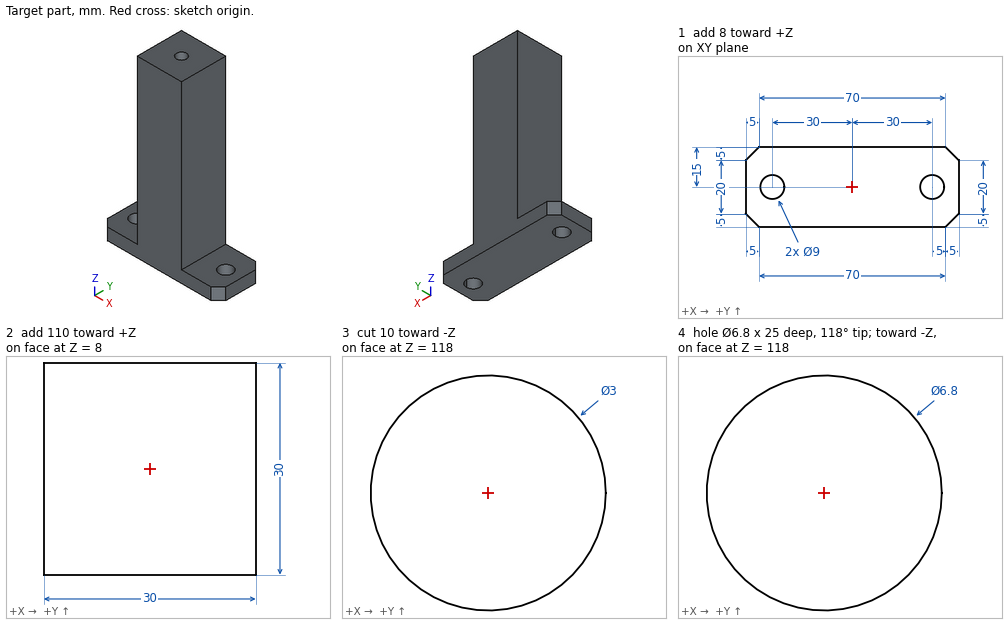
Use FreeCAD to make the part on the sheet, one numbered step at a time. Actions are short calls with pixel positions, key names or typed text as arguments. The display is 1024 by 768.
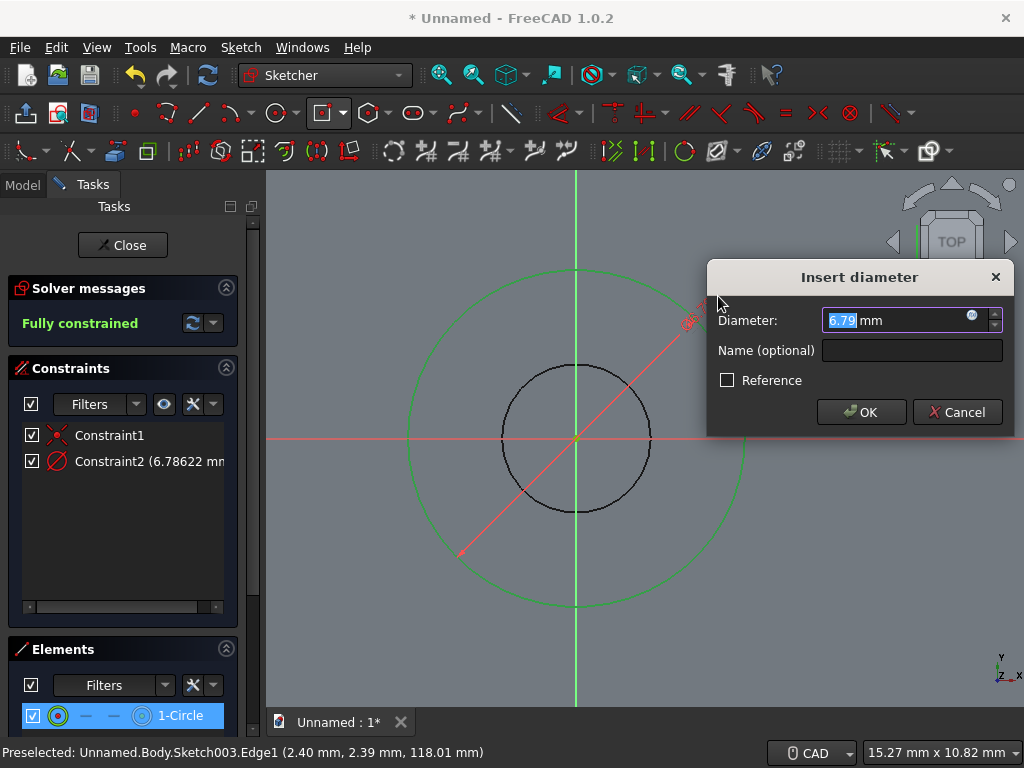
text(6.8)
key(Return)
key(Escape)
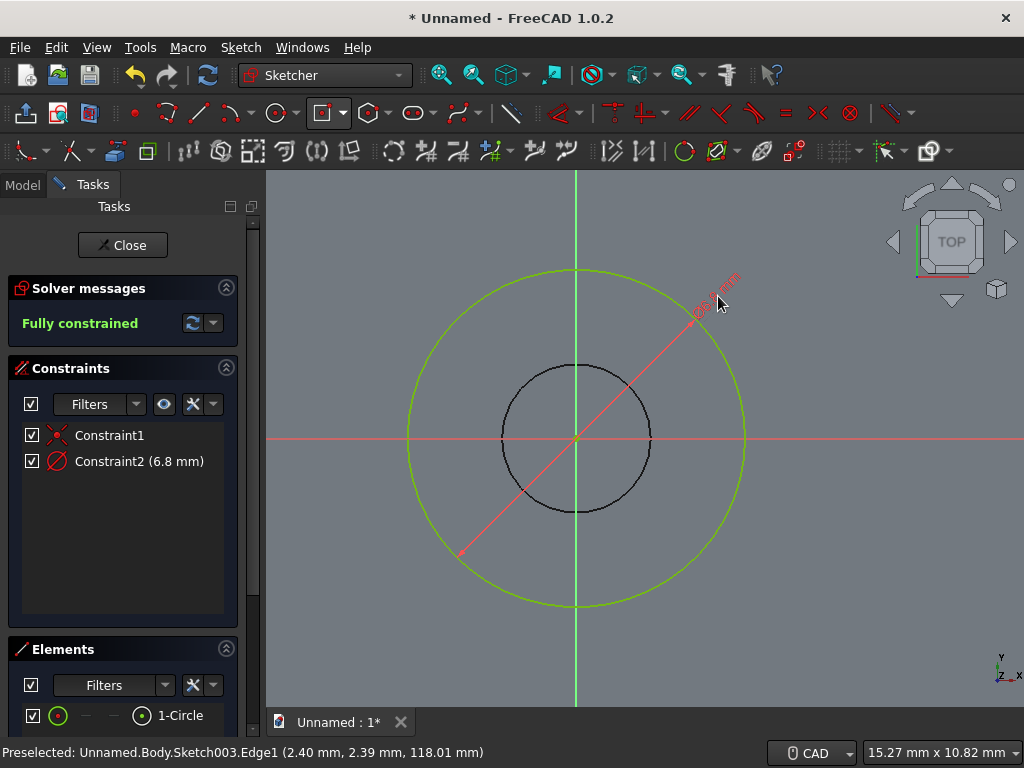
click(123, 245)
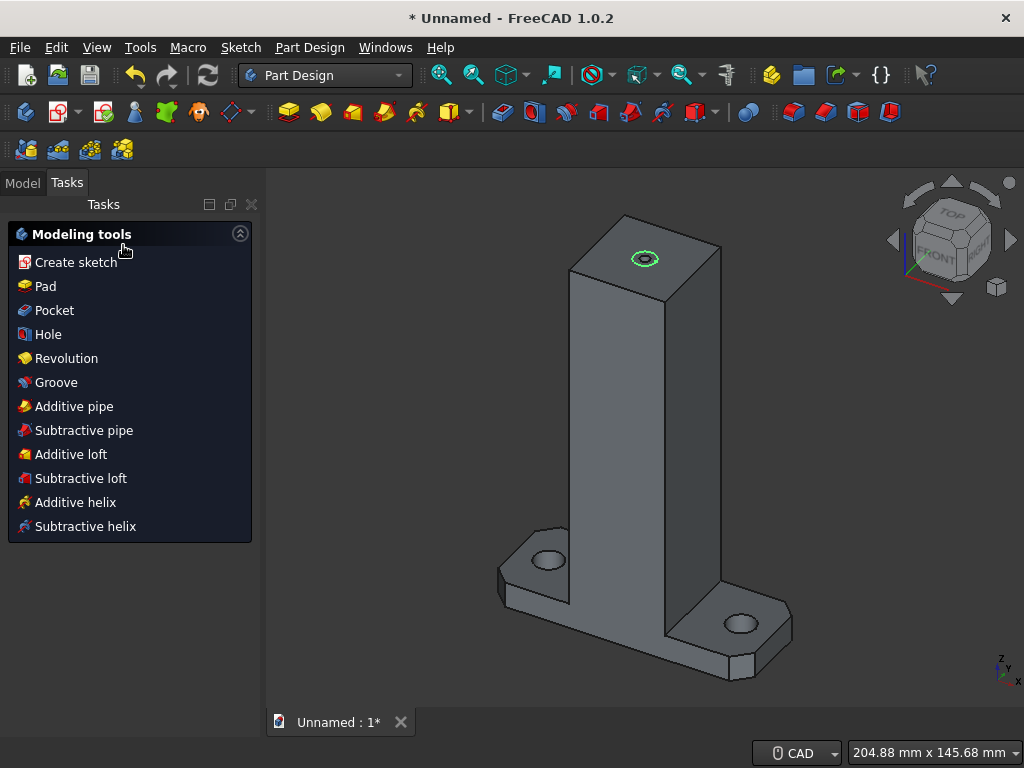
click(536, 112)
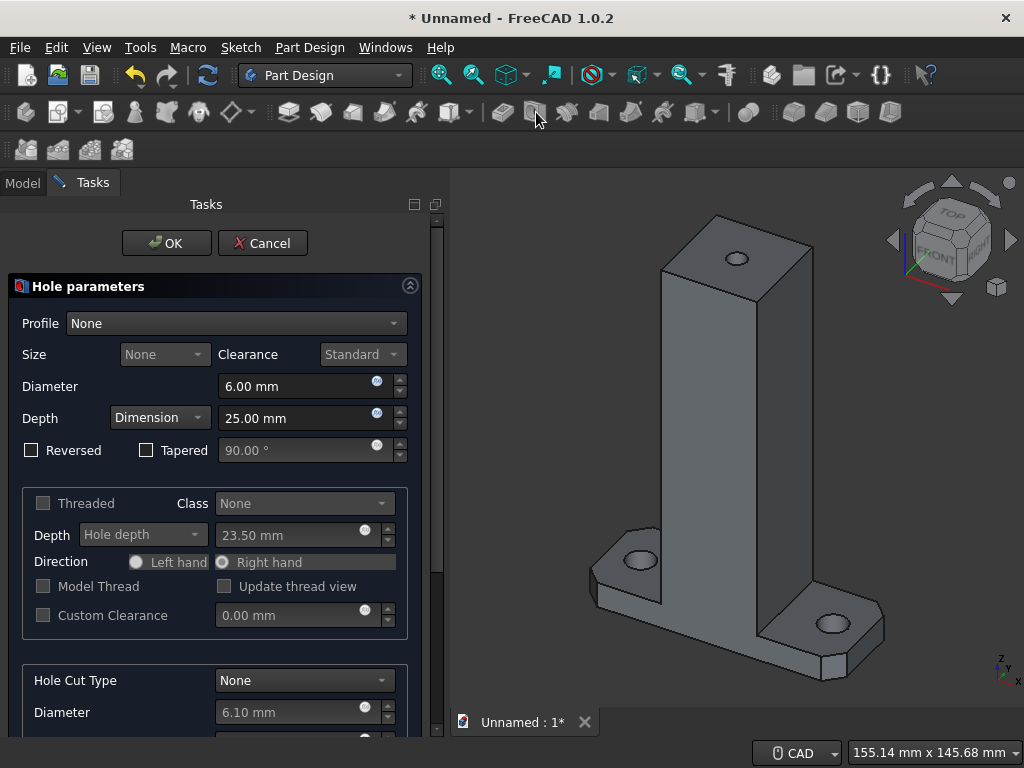
triple_click(305, 386)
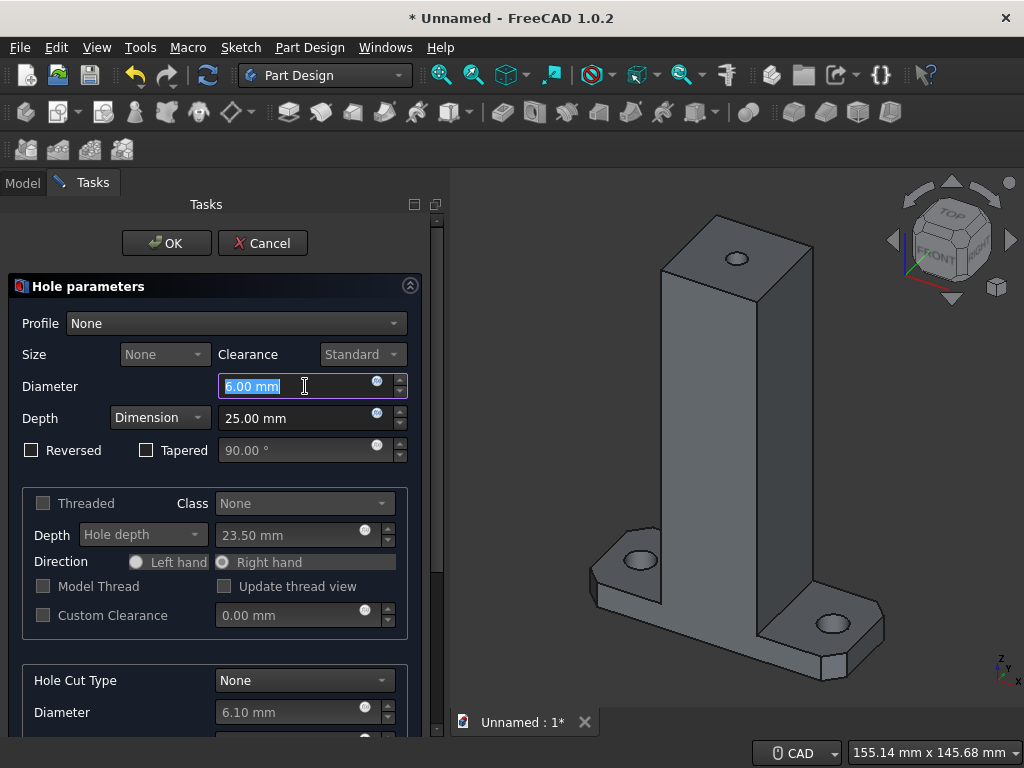
text(6.8)
key(Tab)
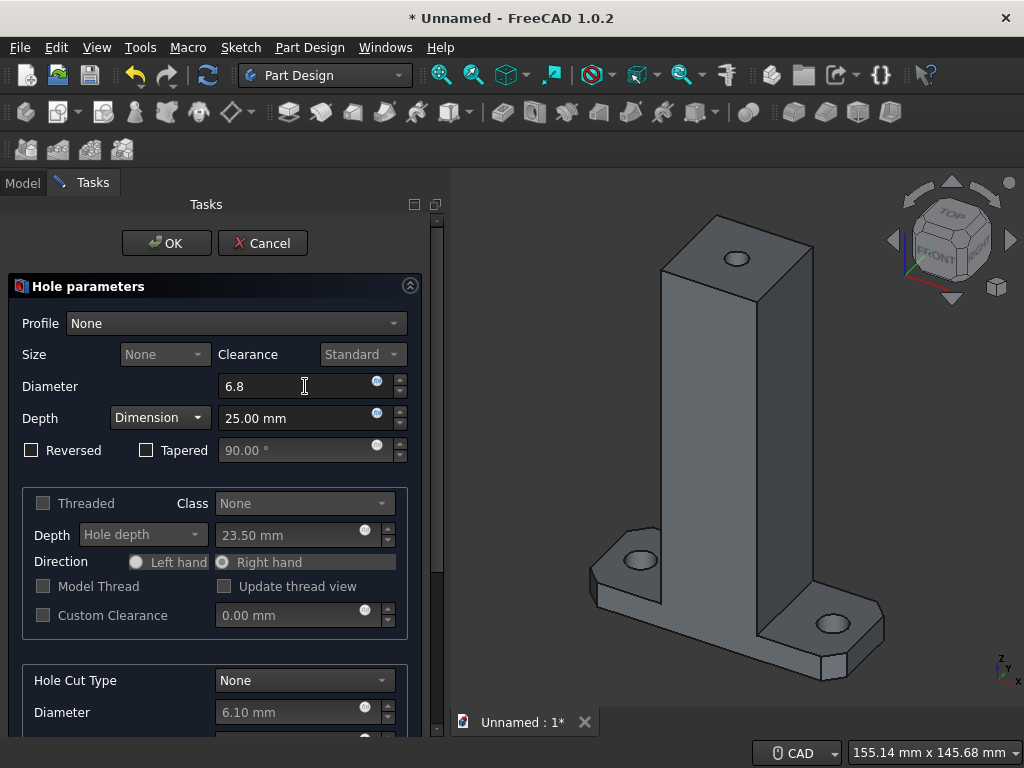
triple_click(305, 418)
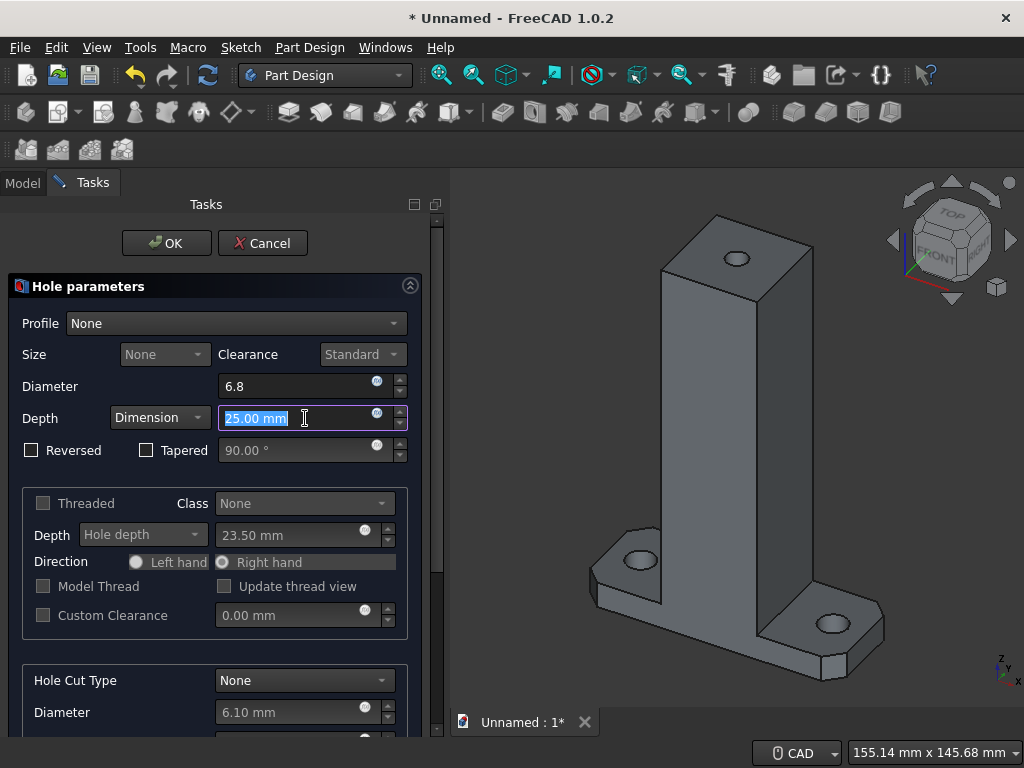
text(25)
key(Tab)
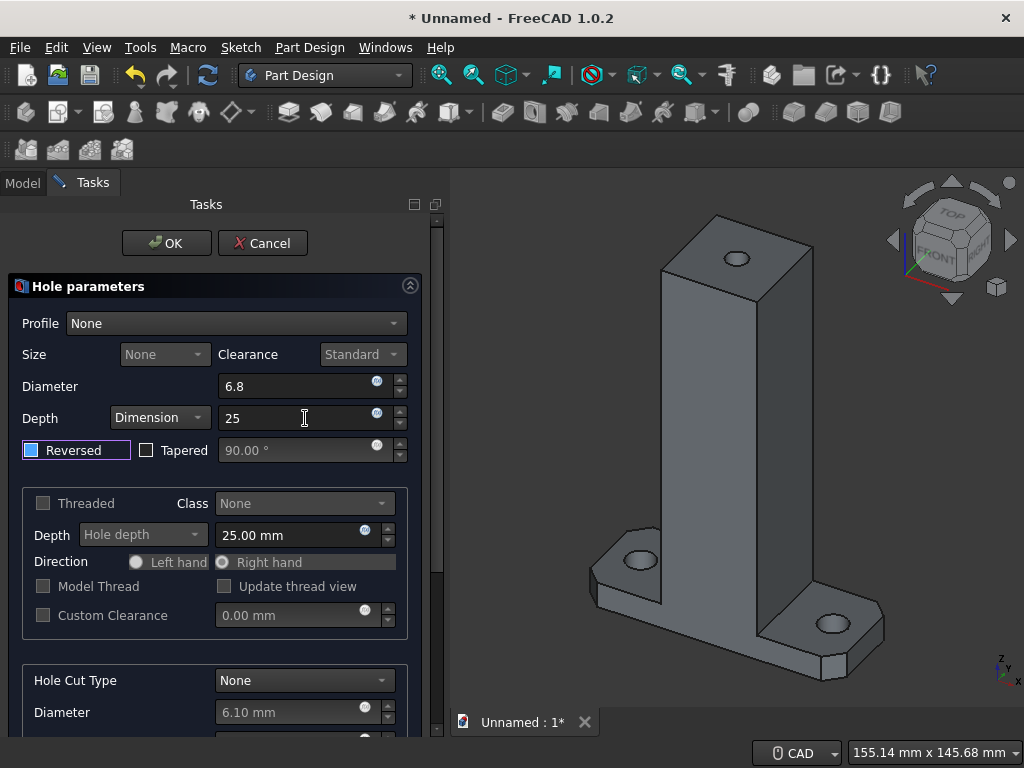
click(167, 243)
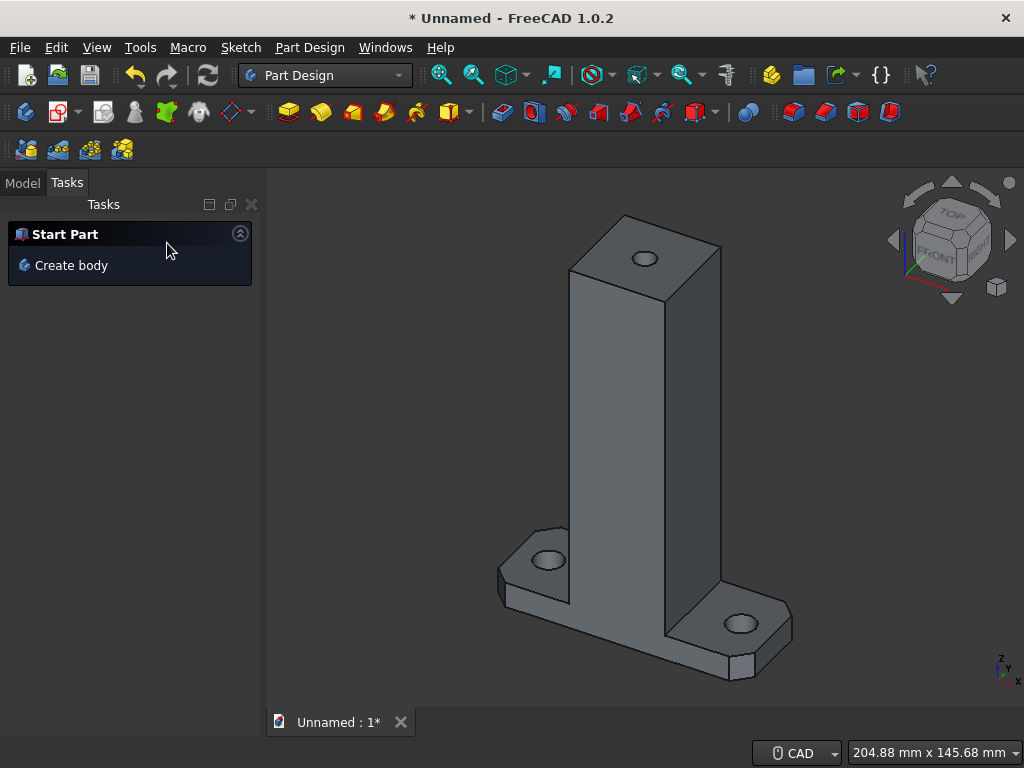
key(0)